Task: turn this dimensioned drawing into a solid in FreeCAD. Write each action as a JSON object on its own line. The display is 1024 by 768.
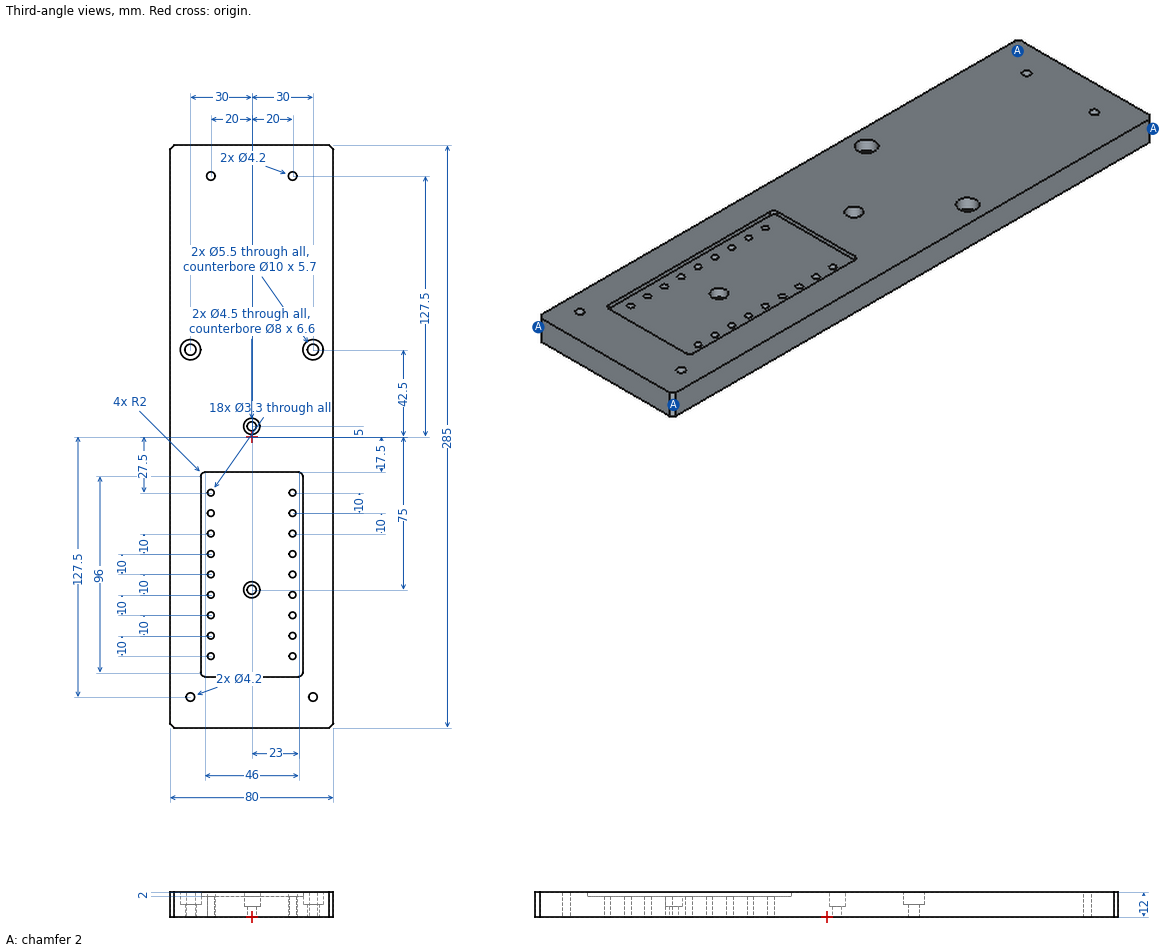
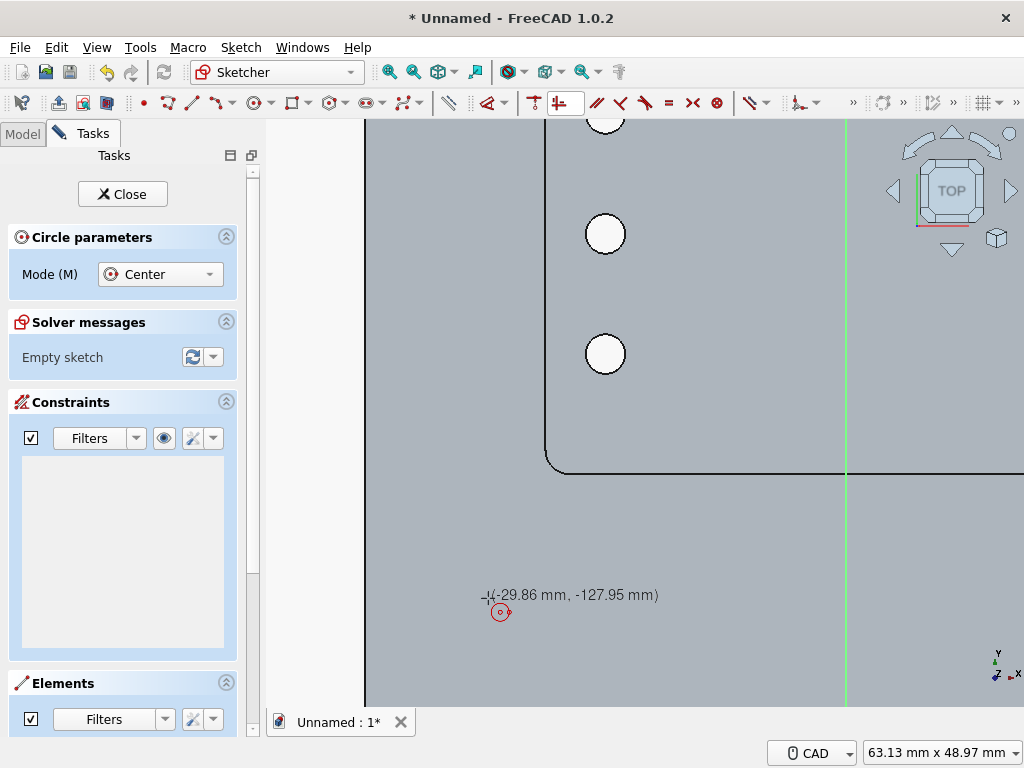
{"action": "scroll", "coordinate": [488, 600], "scroll_direction": "down", "scroll_amount": 7}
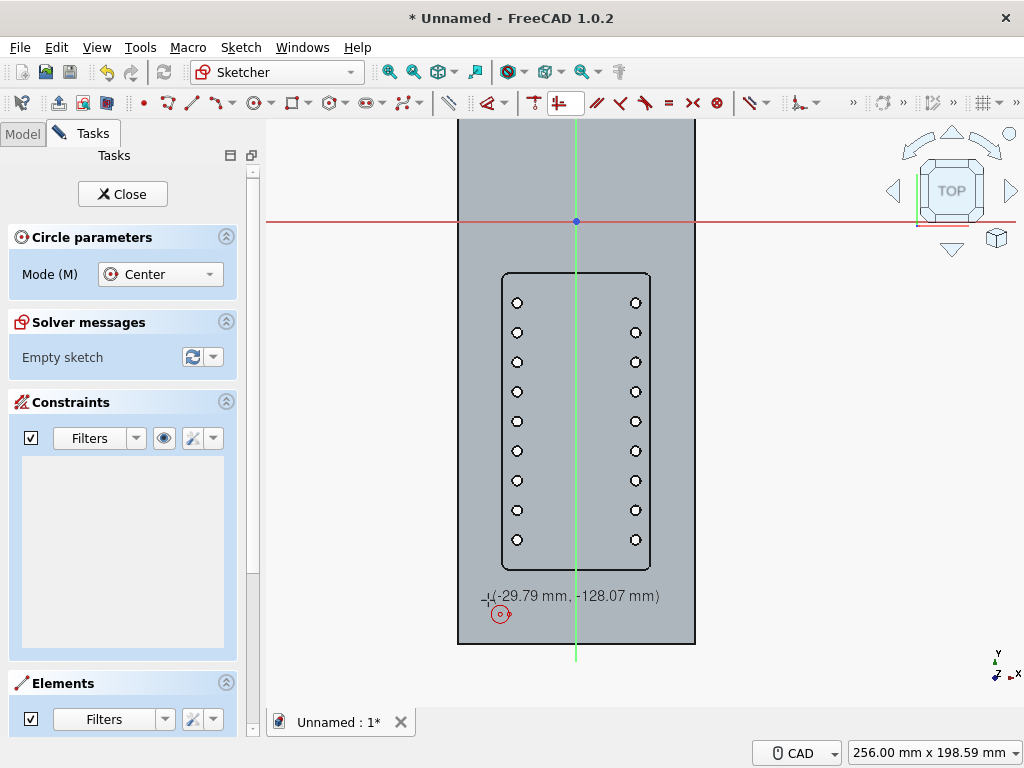
{"action": "left_click", "coordinate": [488, 599]}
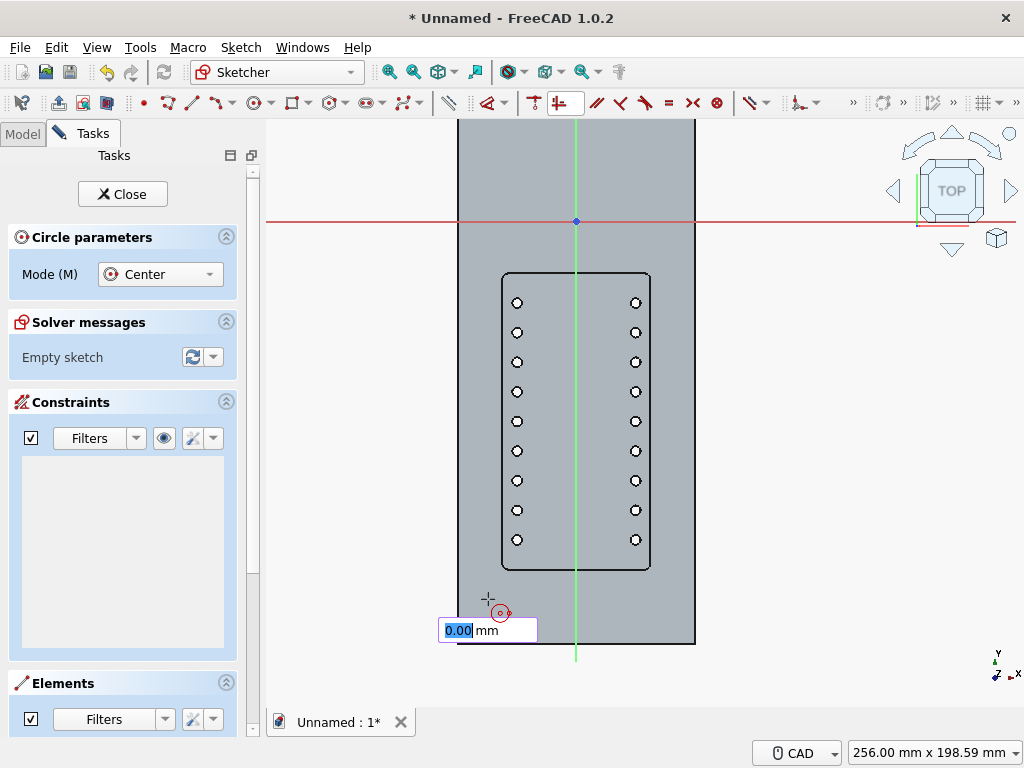
{"action": "scroll", "coordinate": [492, 595], "scroll_direction": "up", "scroll_amount": 5}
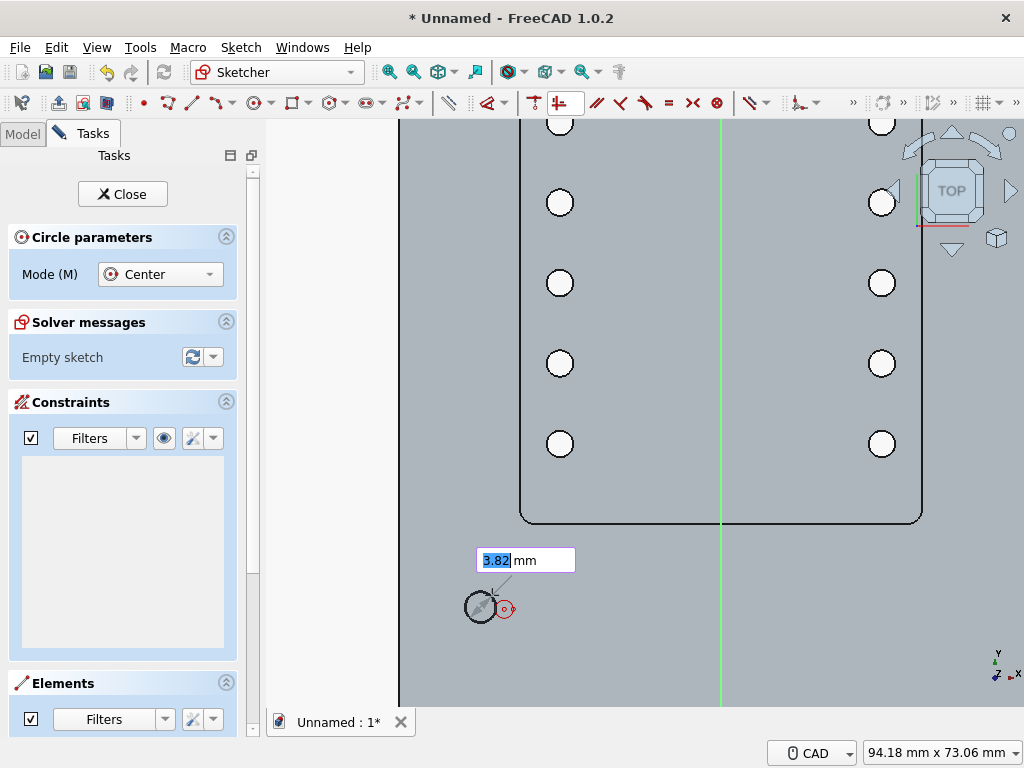
{"action": "left_click", "coordinate": [491, 593]}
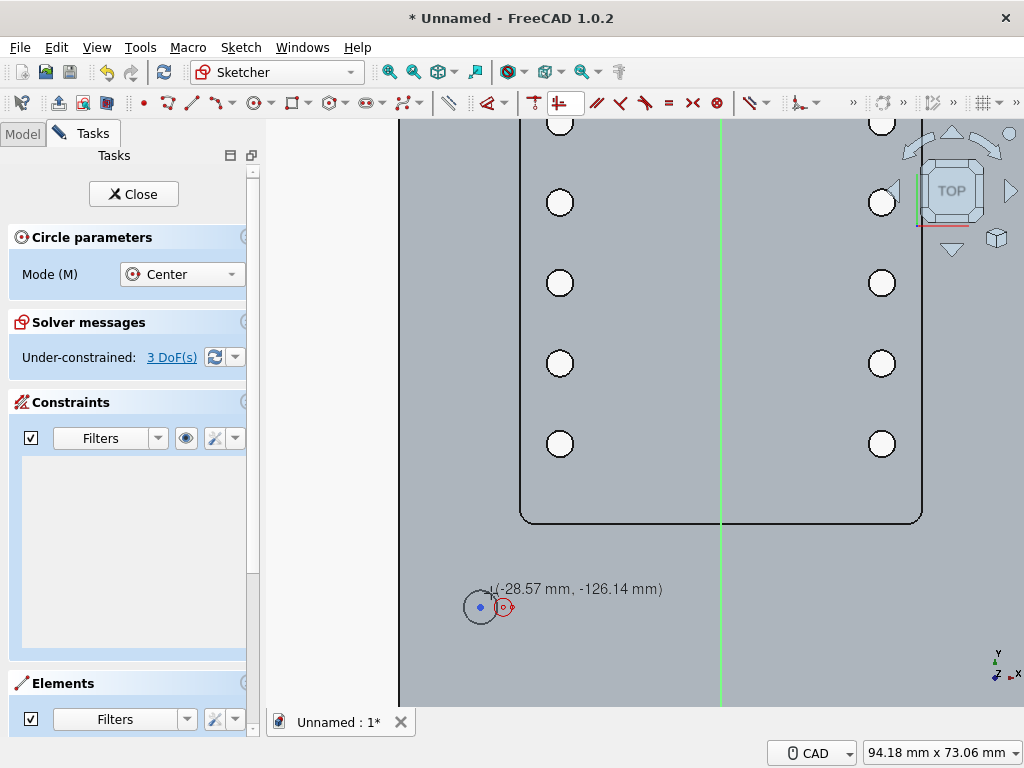
{"action": "scroll", "coordinate": [492, 595], "scroll_direction": "down", "scroll_amount": 5}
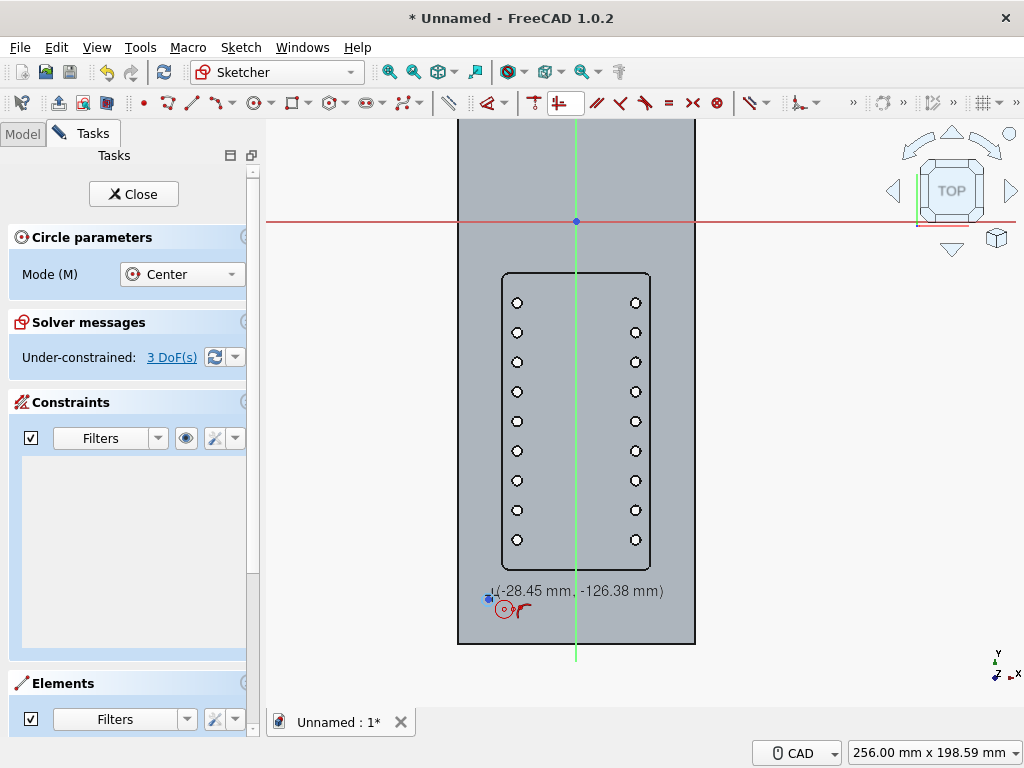
{"action": "scroll", "coordinate": [665, 599], "scroll_direction": "up", "scroll_amount": 7}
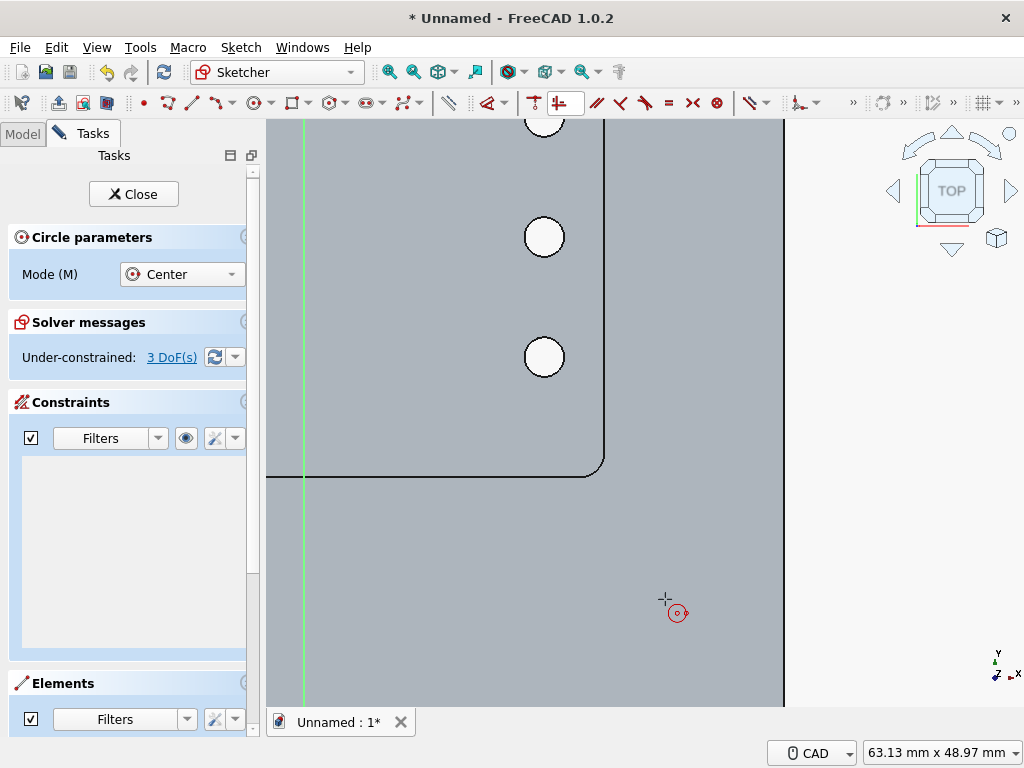
{"action": "scroll", "coordinate": [666, 599], "scroll_direction": "down", "scroll_amount": 7}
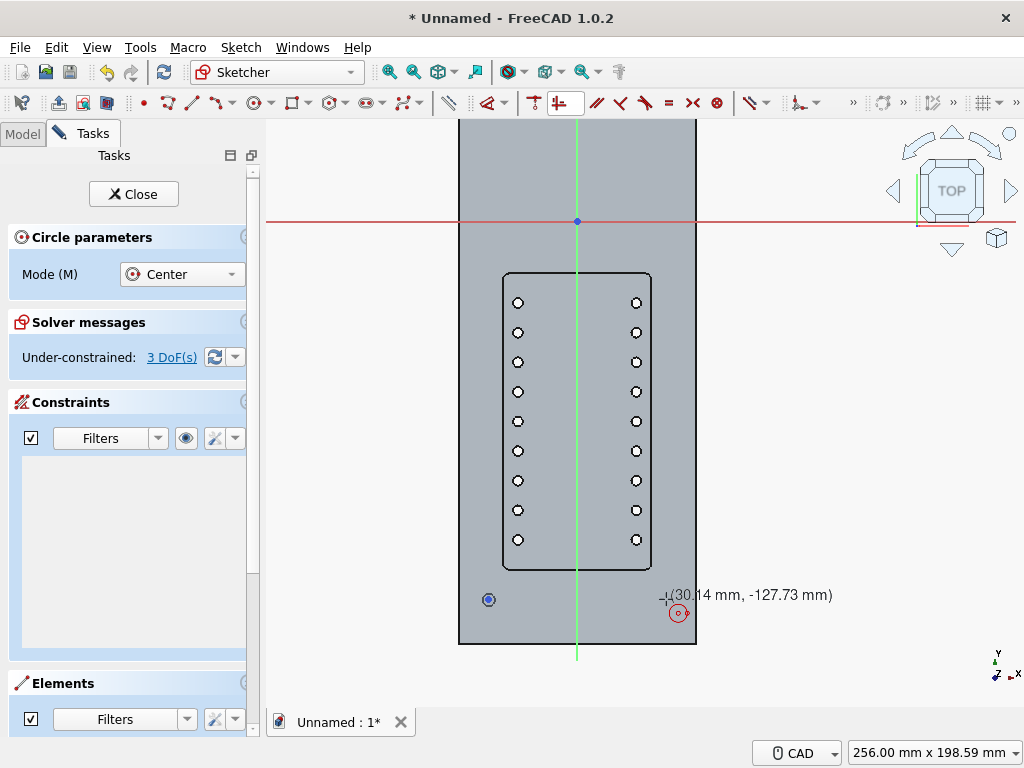
{"action": "left_click", "coordinate": [666, 599]}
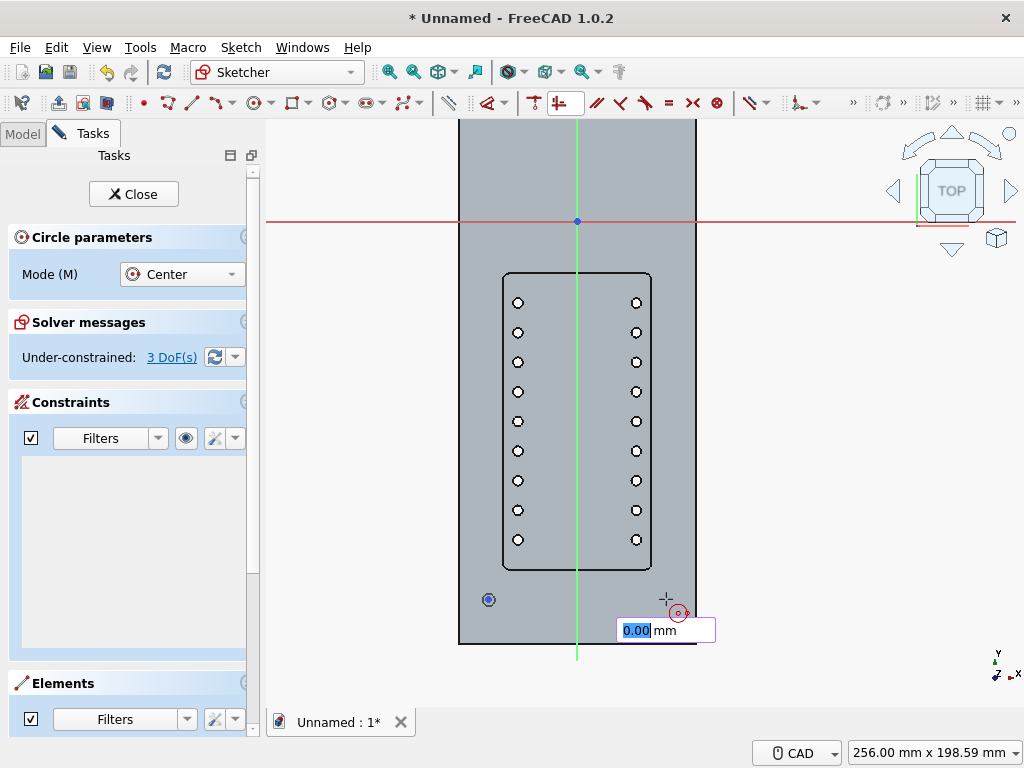
{"action": "scroll", "coordinate": [670, 595], "scroll_direction": "up", "scroll_amount": 5}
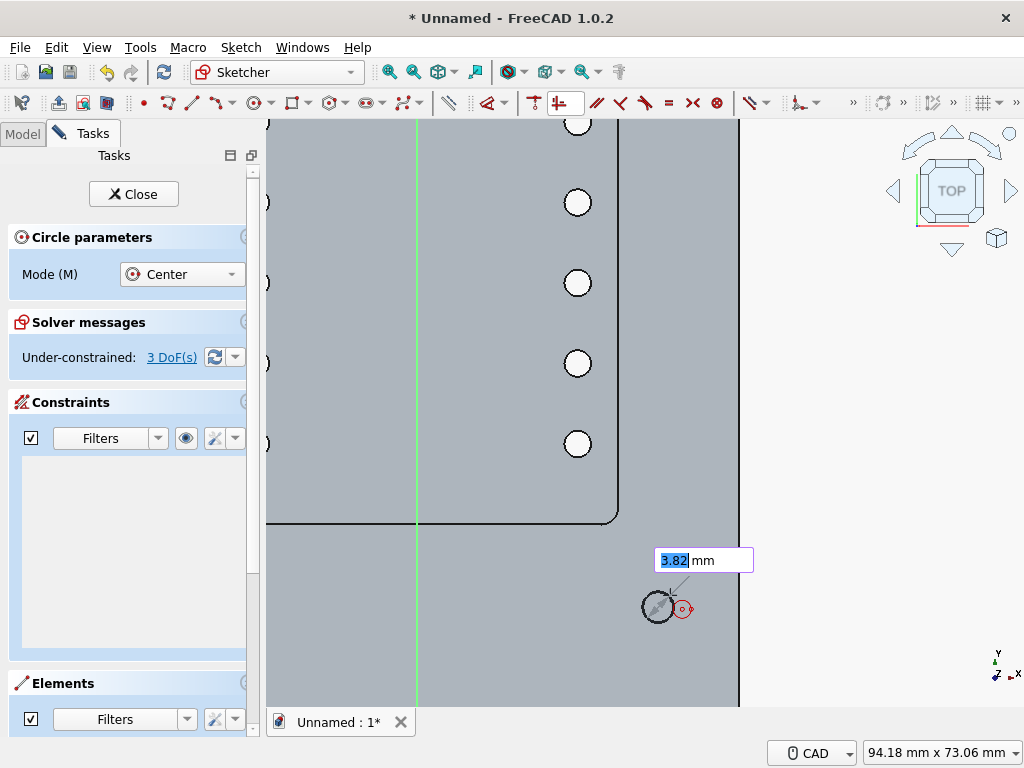
{"action": "left_click", "coordinate": [670, 593]}
{"action": "key", "text": "Escape"}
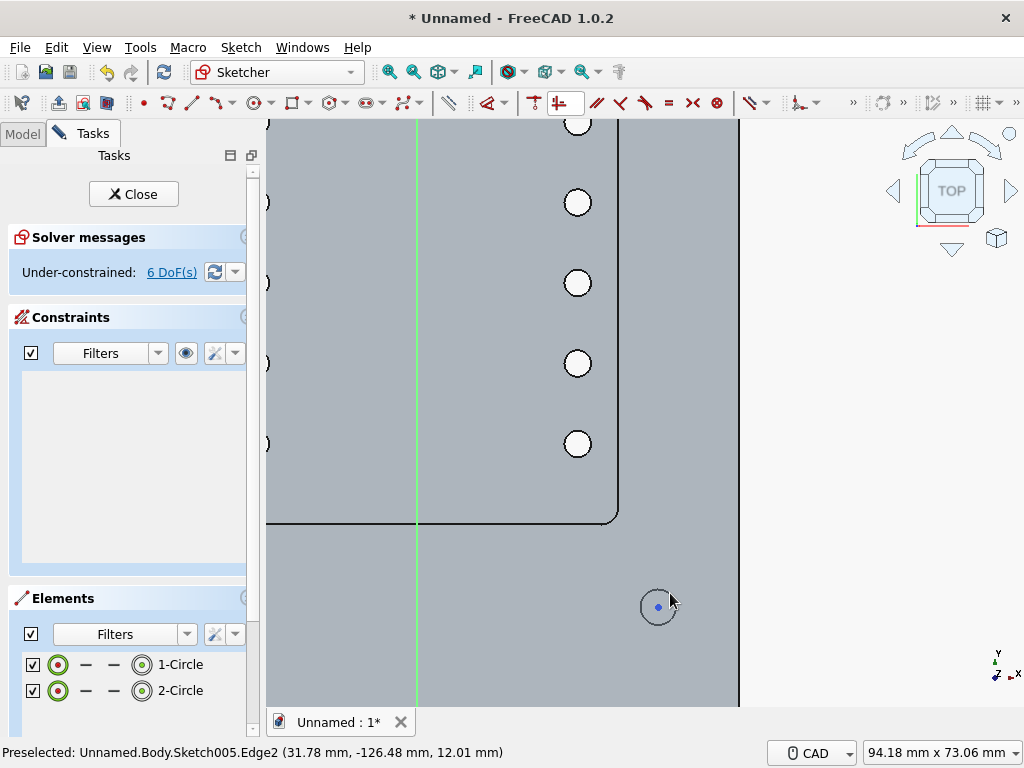
{"action": "scroll", "coordinate": [669, 595], "scroll_direction": "down", "scroll_amount": 5}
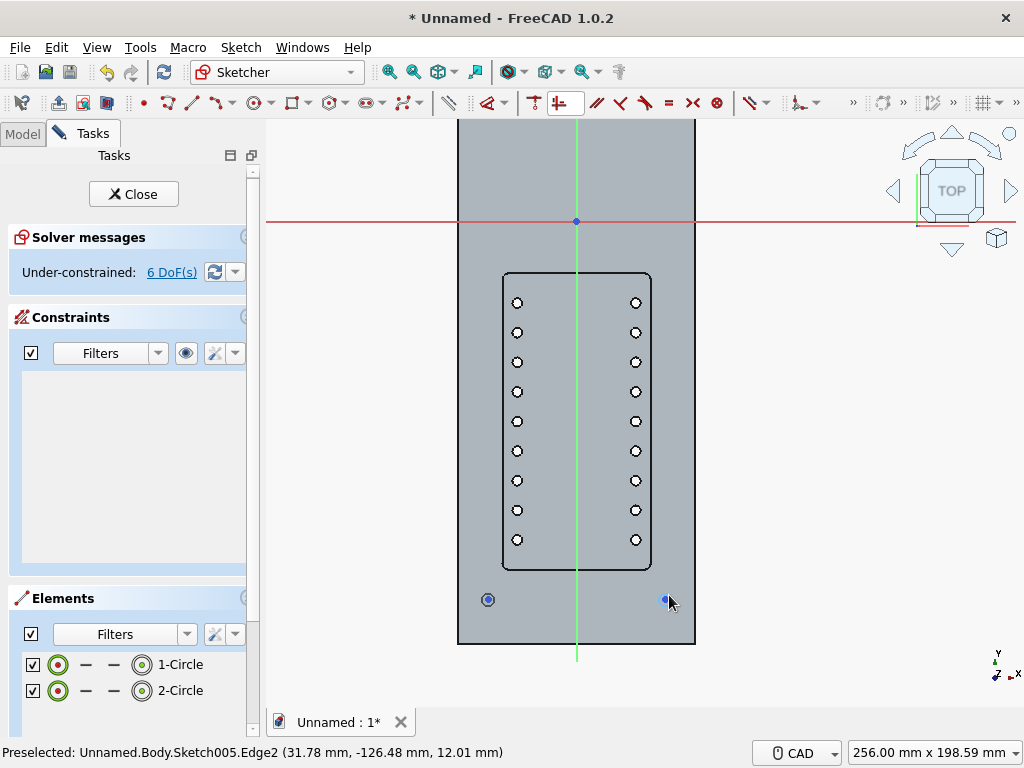
{"action": "scroll", "coordinate": [492, 596], "scroll_direction": "up", "scroll_amount": 5}